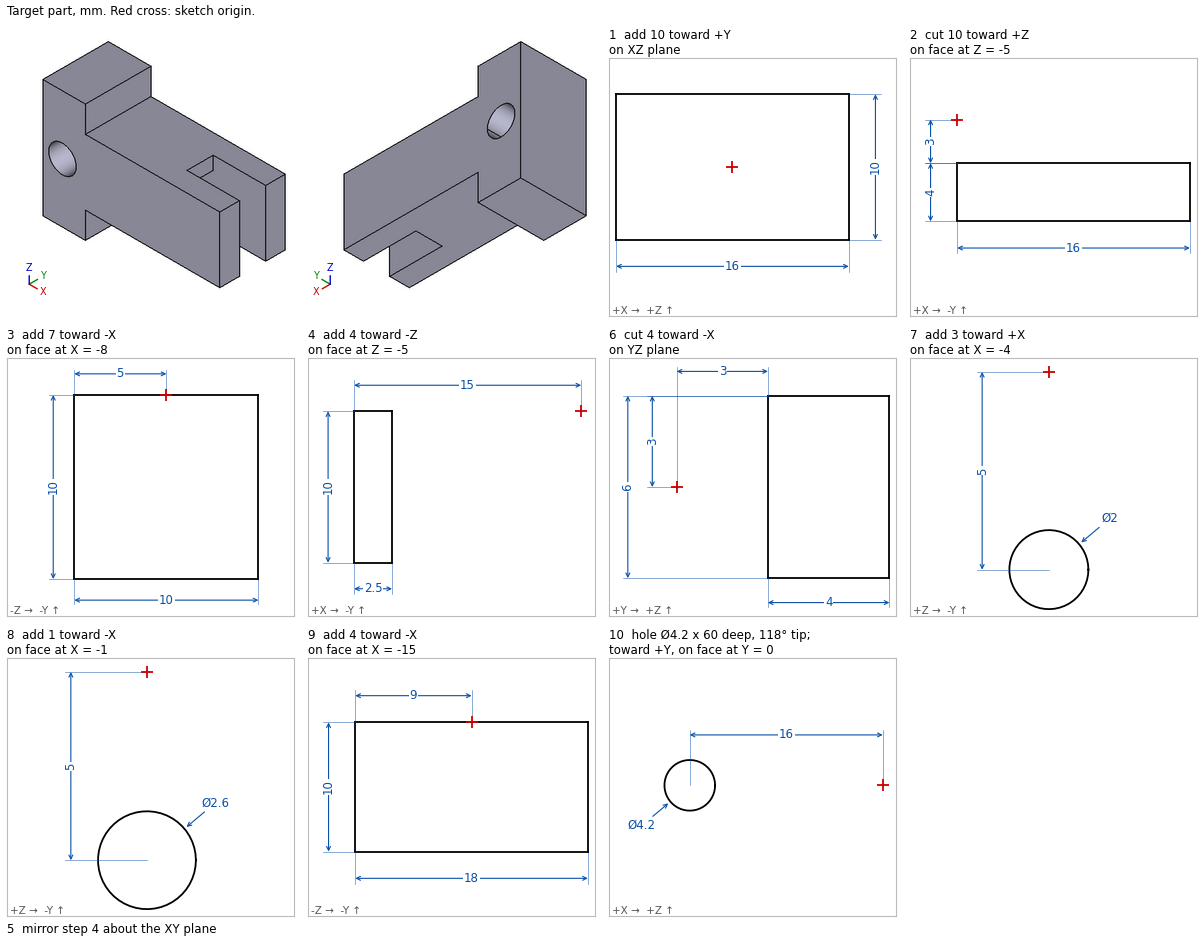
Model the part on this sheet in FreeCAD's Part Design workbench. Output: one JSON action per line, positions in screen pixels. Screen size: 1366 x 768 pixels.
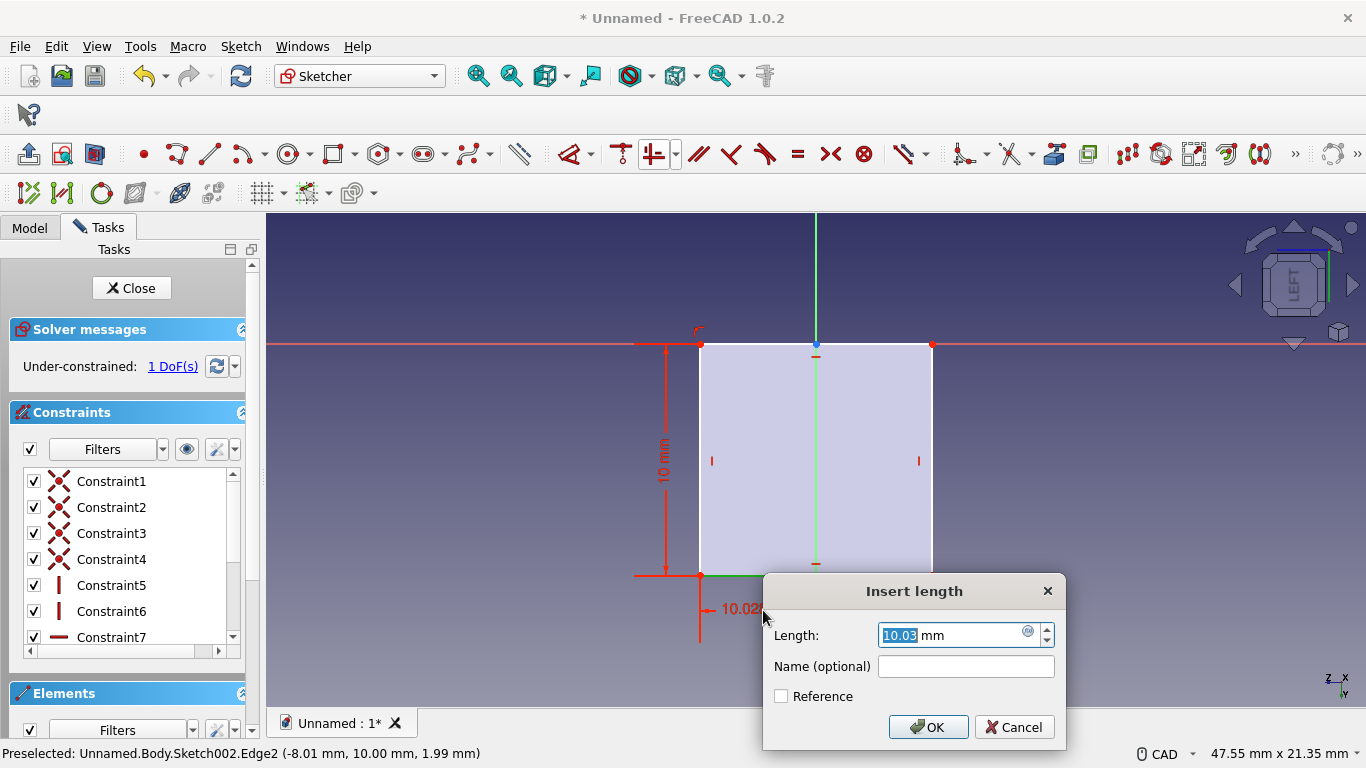
{"action": "type", "text": "10"}
{"action": "key", "text": "Return"}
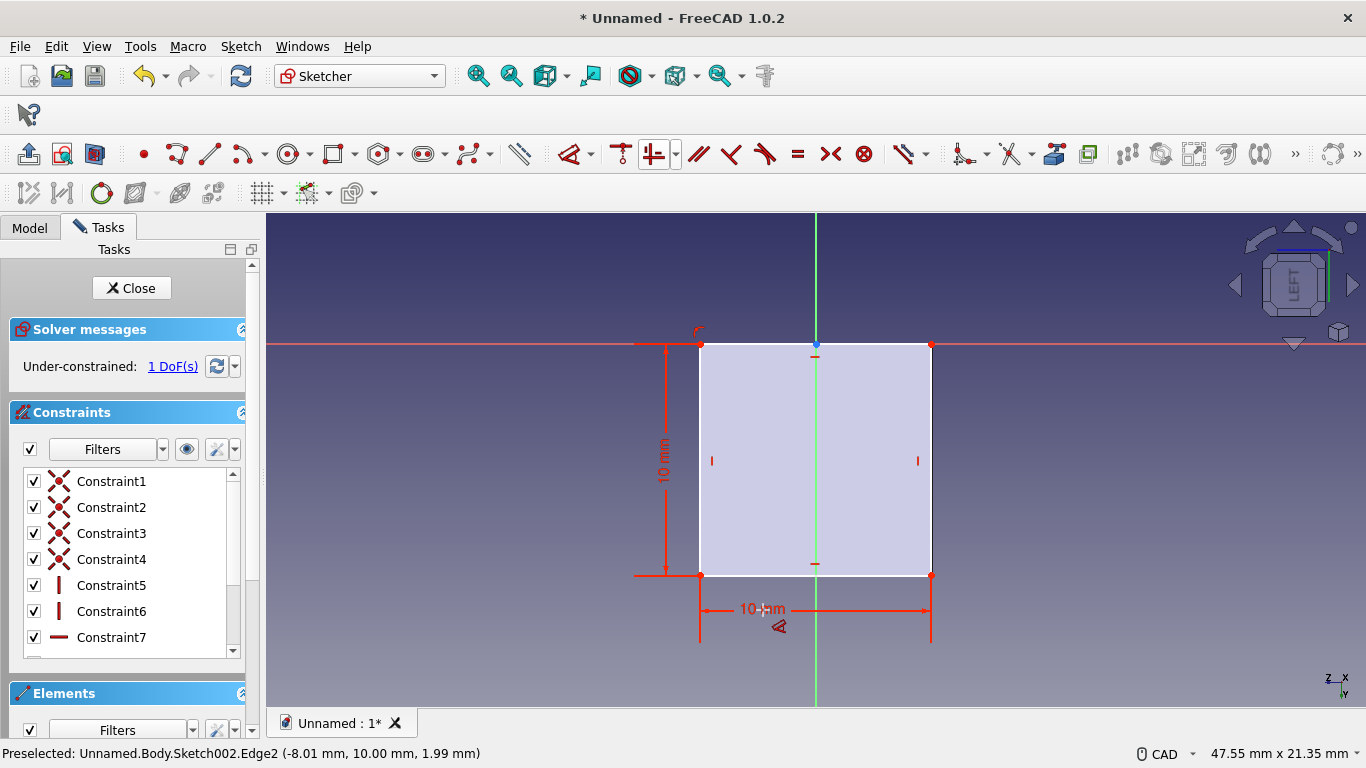
{"action": "left_click", "coordinate": [700, 344]}
{"action": "left_click", "coordinate": [758, 310]}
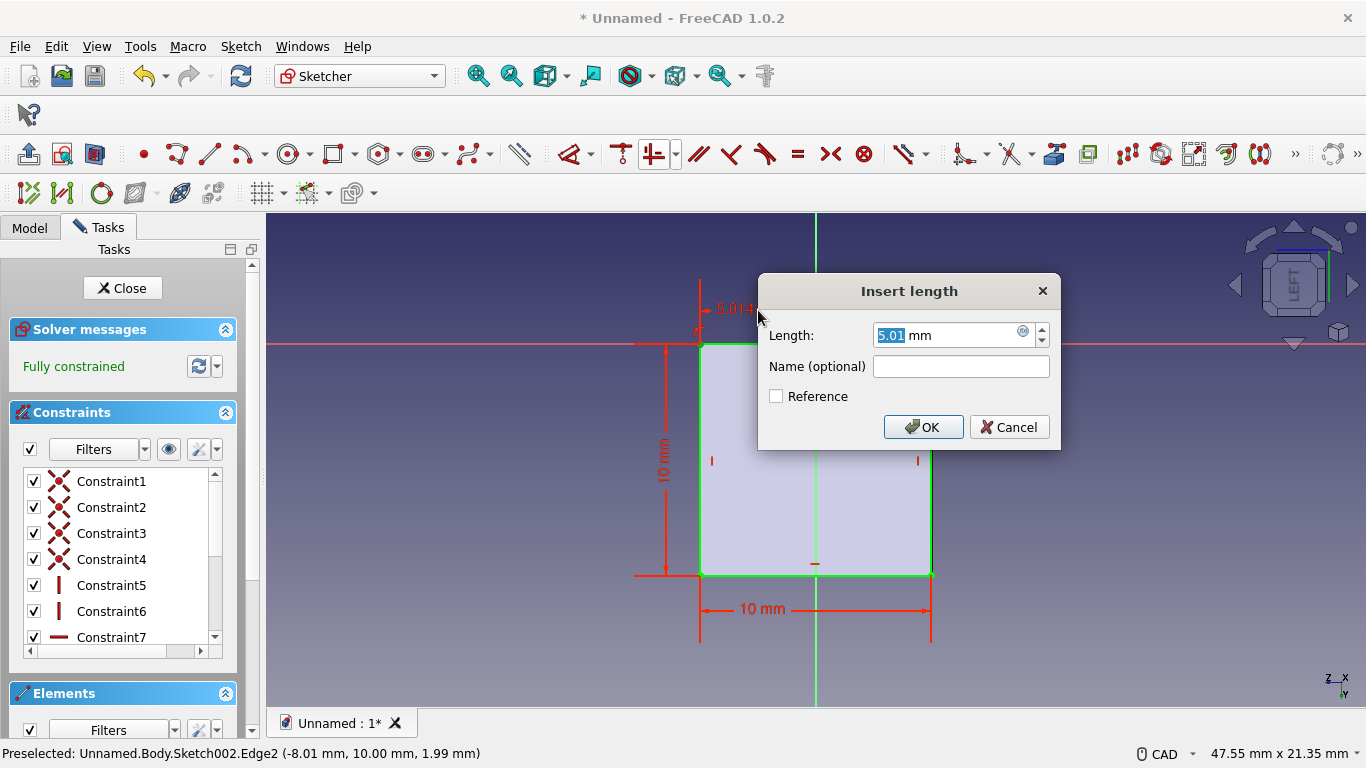
{"action": "type", "text": "5"}
{"action": "key", "text": "Return"}
{"action": "key", "text": "Escape"}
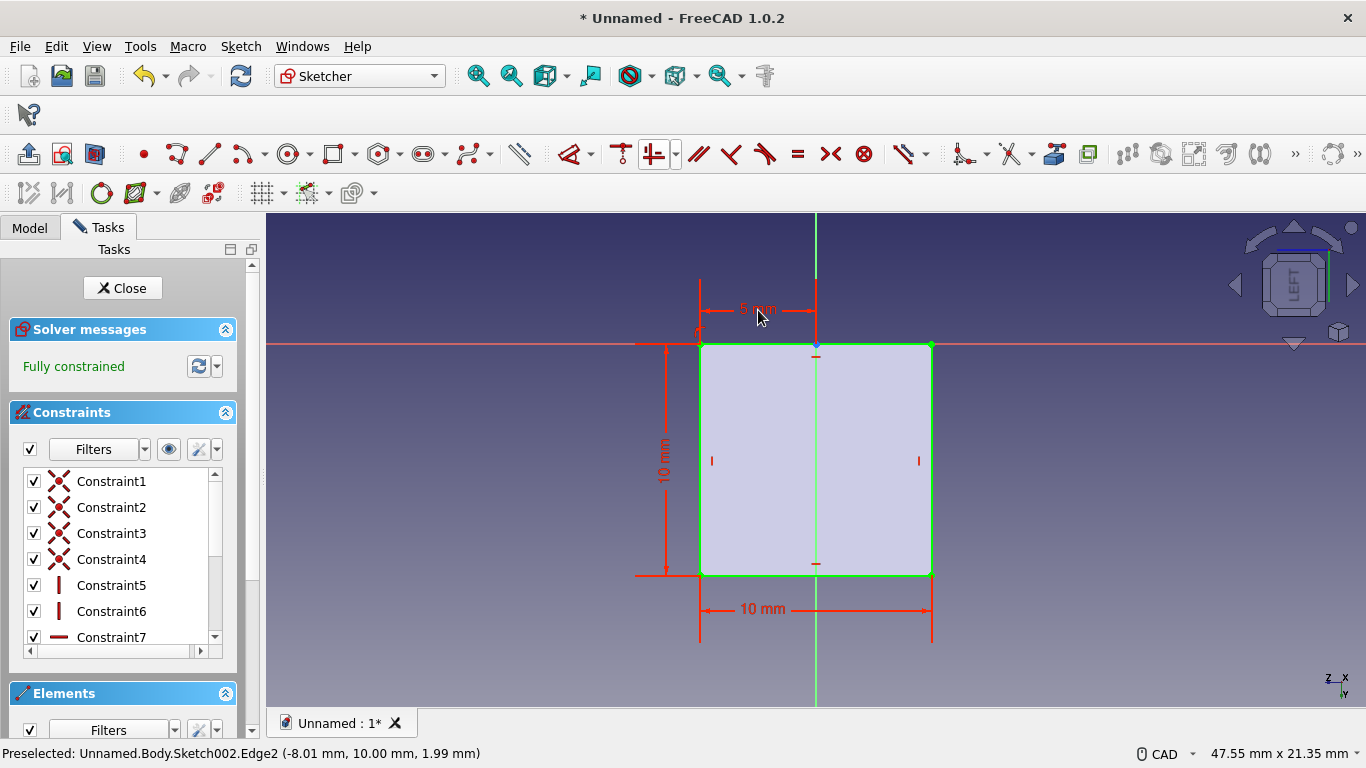
{"action": "left_click", "coordinate": [123, 288]}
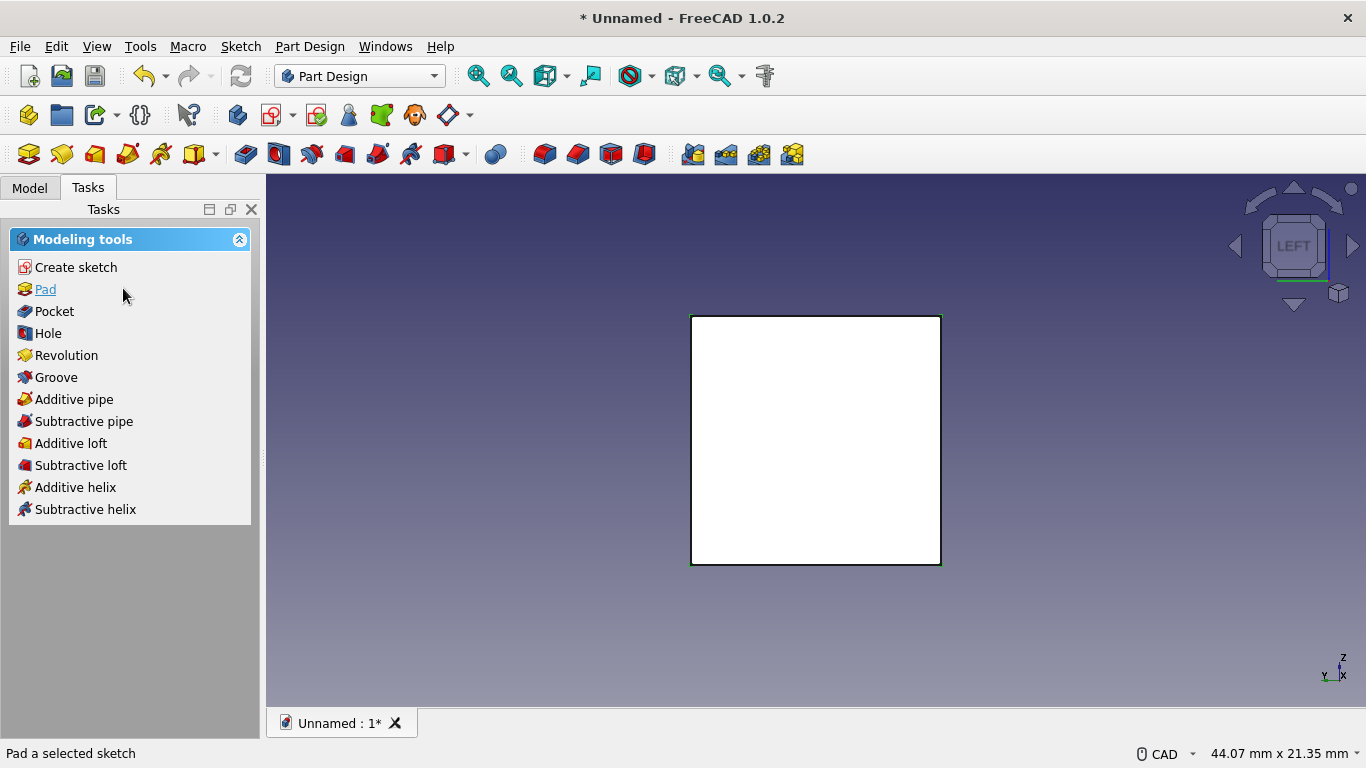
{"action": "left_click", "coordinate": [29, 154]}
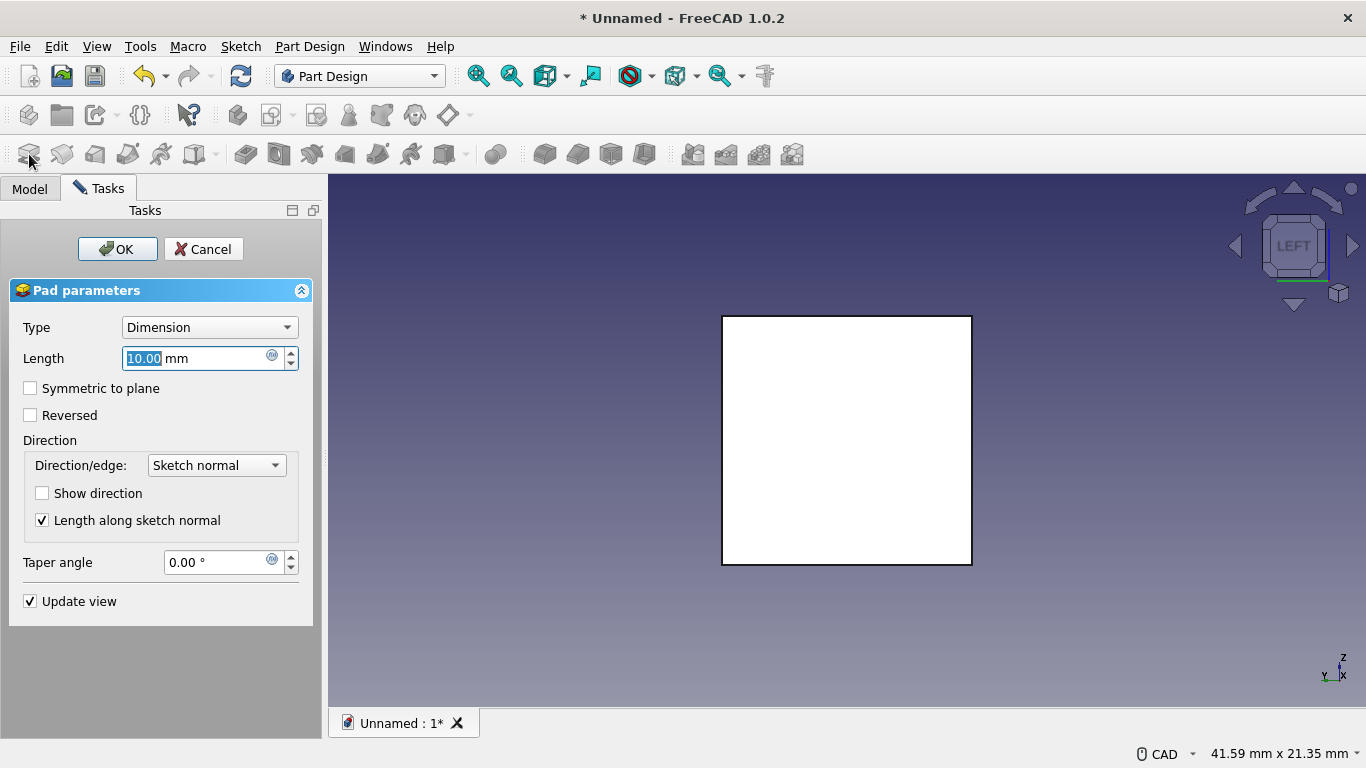
{"action": "type", "text": "7"}
{"action": "key", "text": "Tab"}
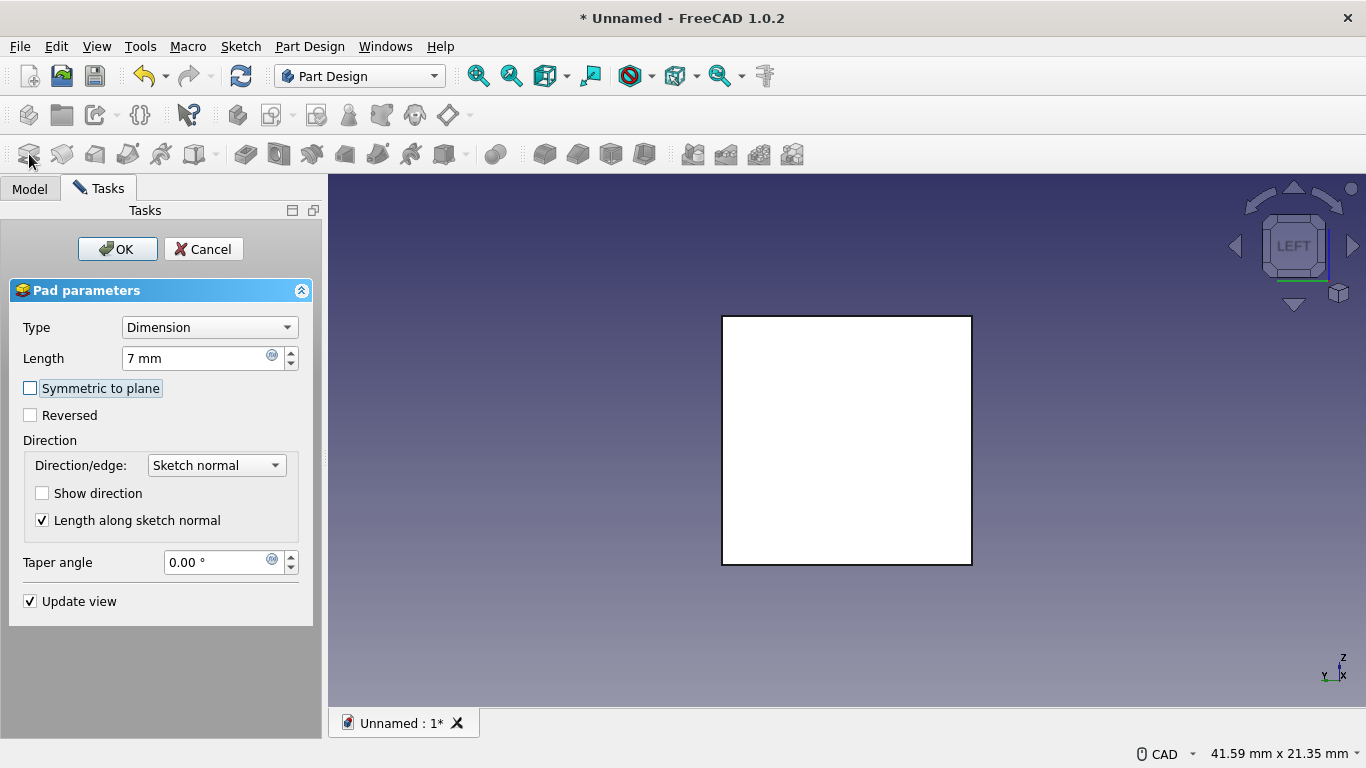
{"action": "left_click", "coordinate": [118, 249]}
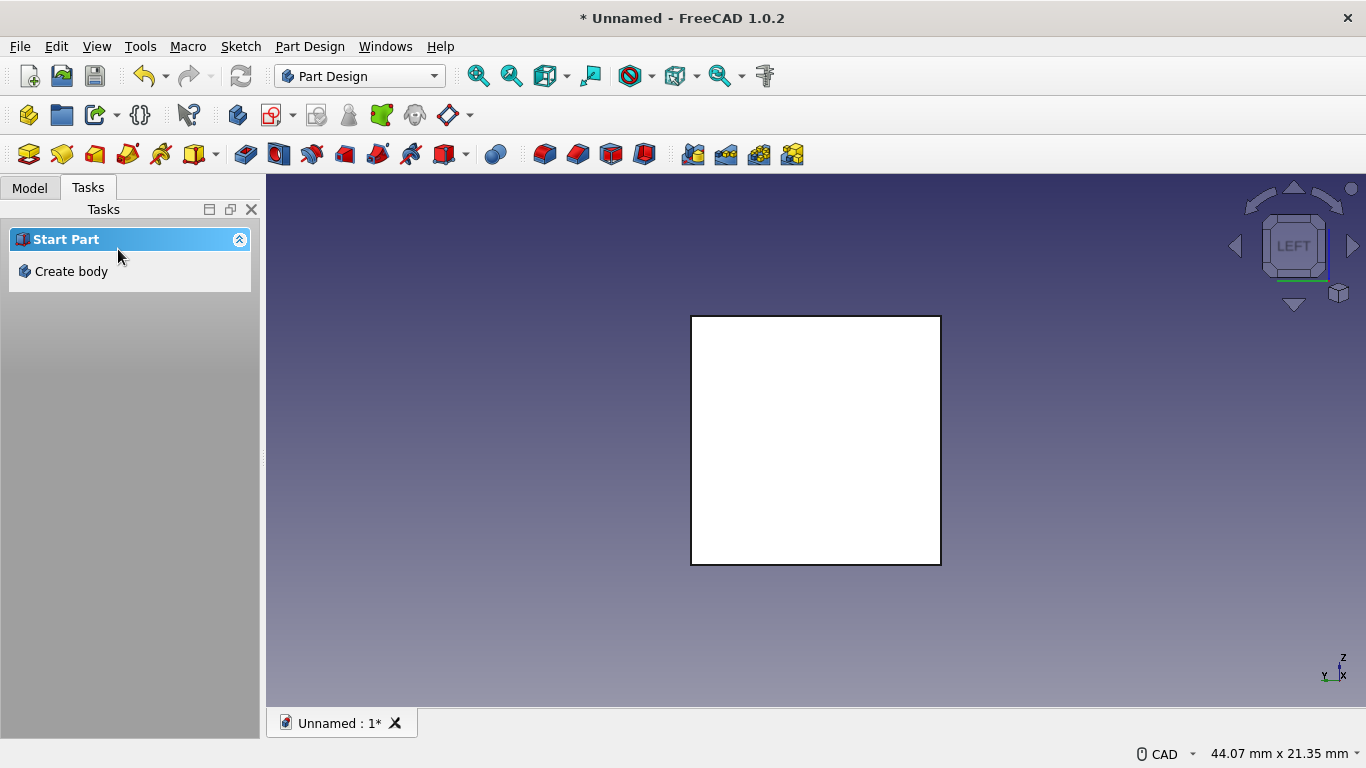
{"action": "key", "text": "5"}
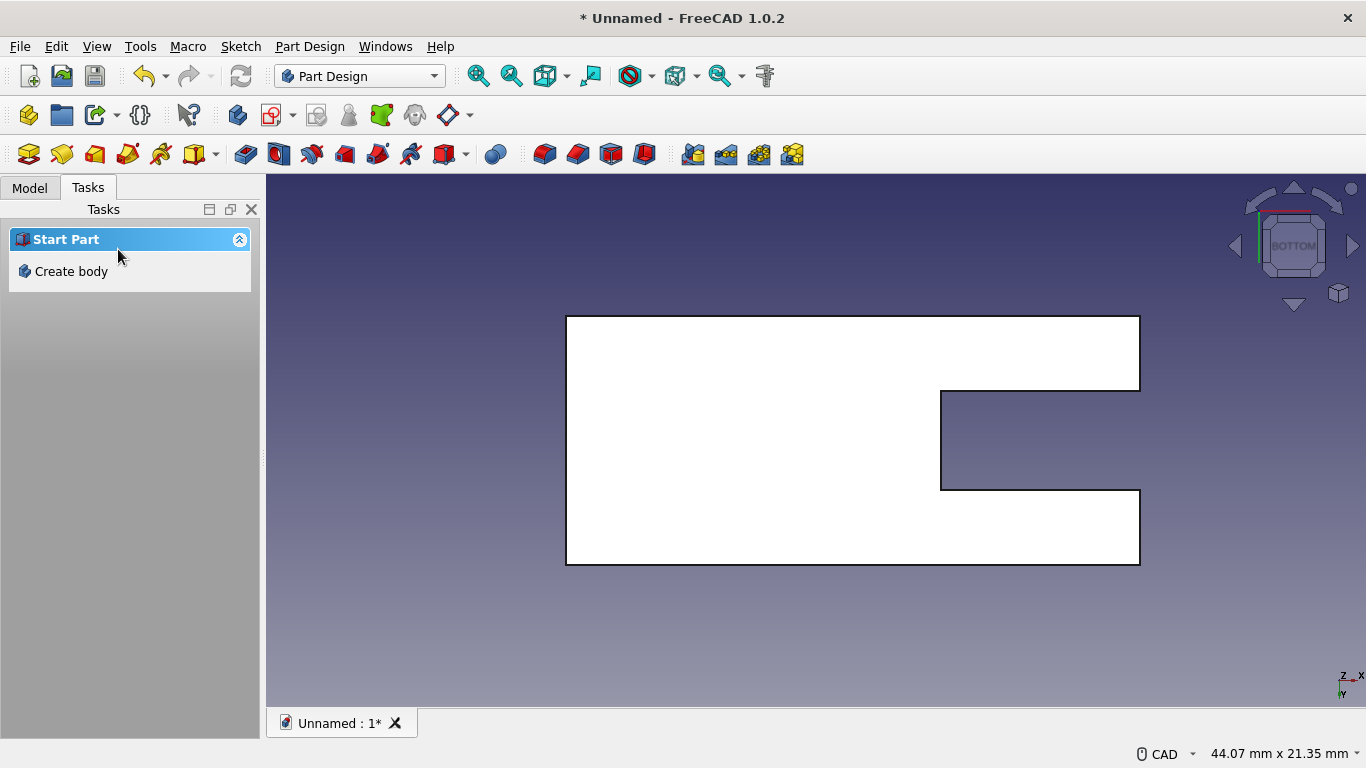
{"action": "left_click", "coordinate": [771, 440]}